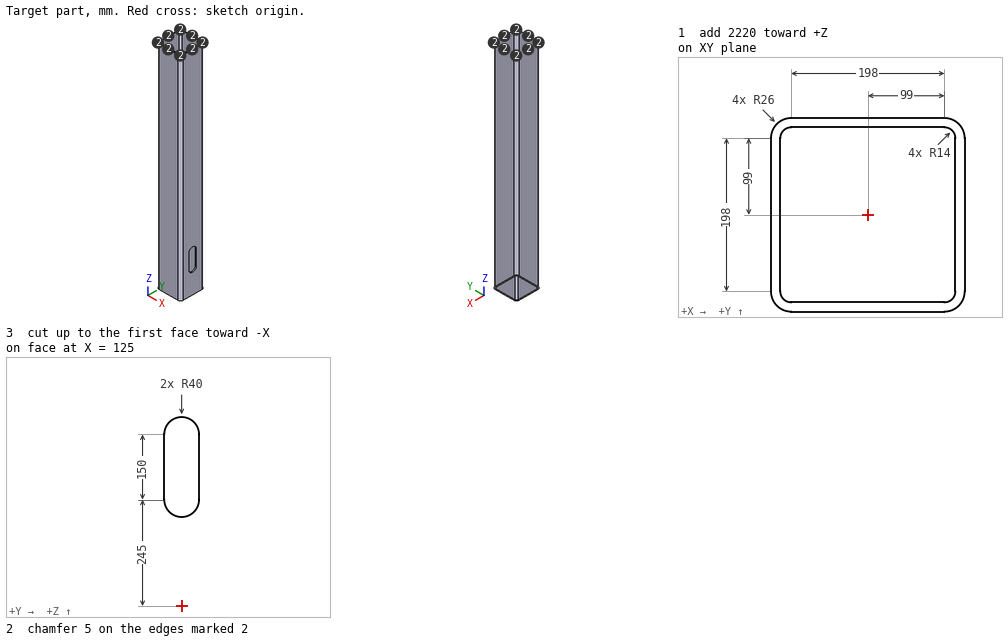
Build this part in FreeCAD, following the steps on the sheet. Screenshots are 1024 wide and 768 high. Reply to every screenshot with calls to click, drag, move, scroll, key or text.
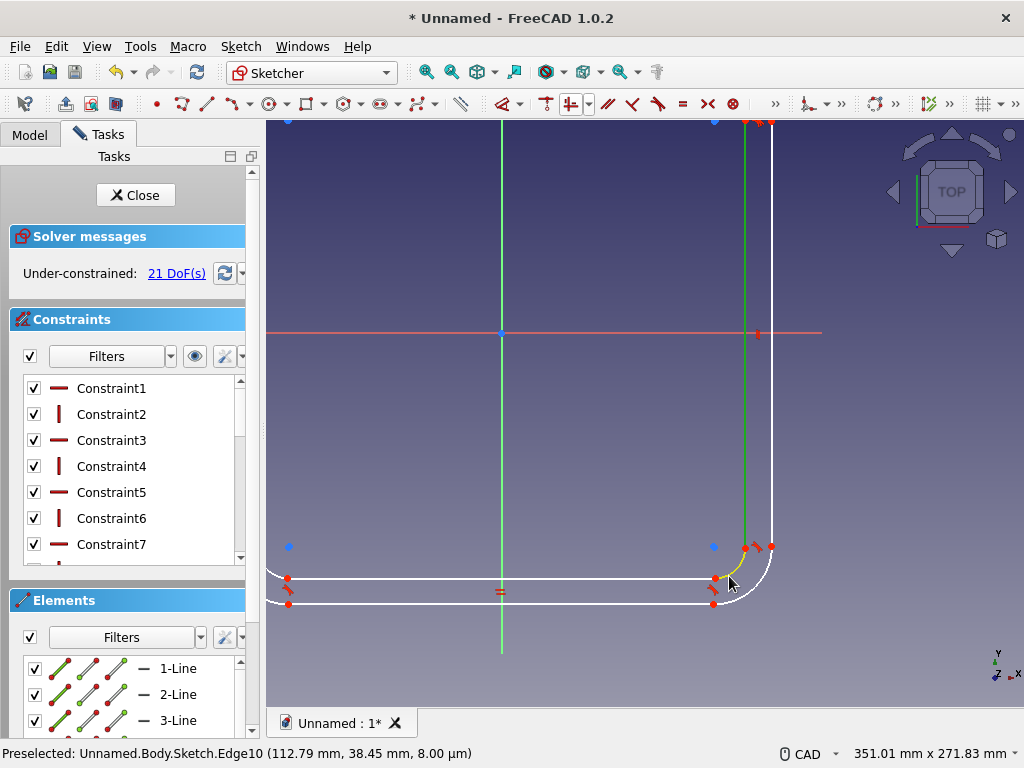
click(729, 575)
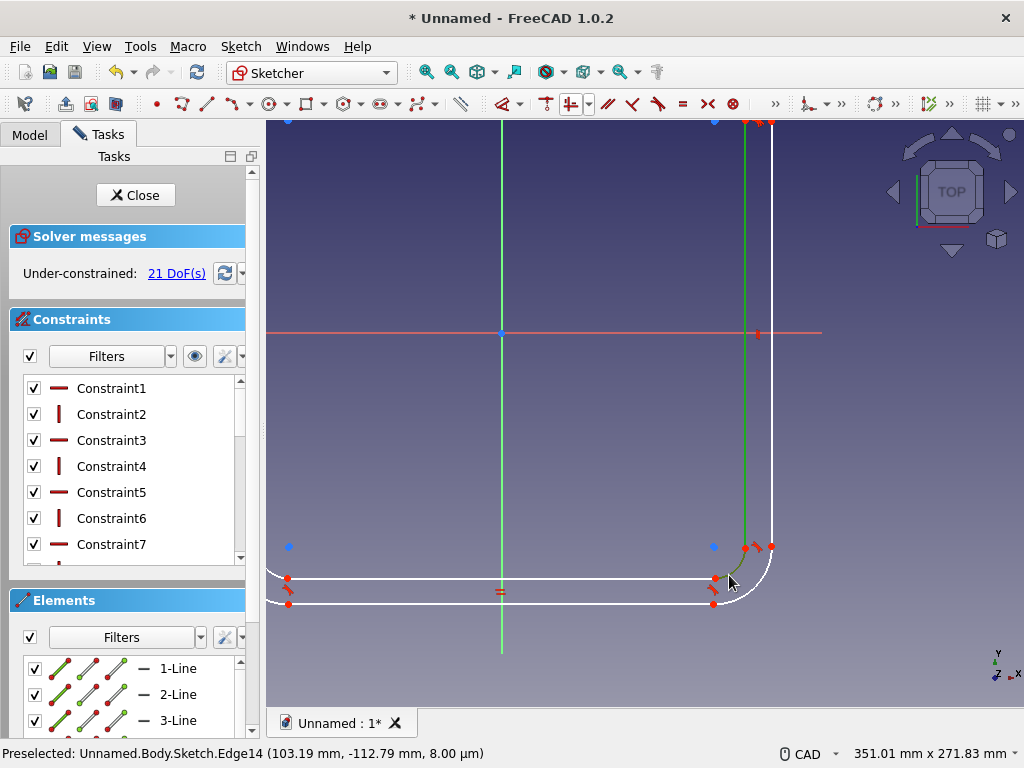
click(658, 104)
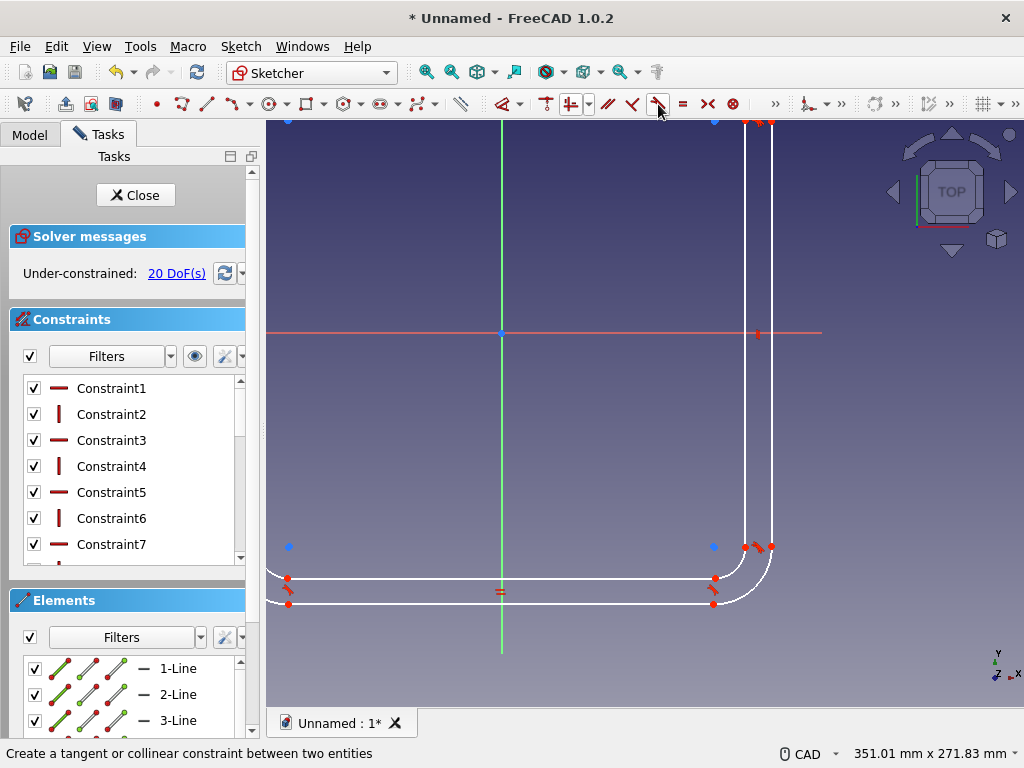
click(587, 579)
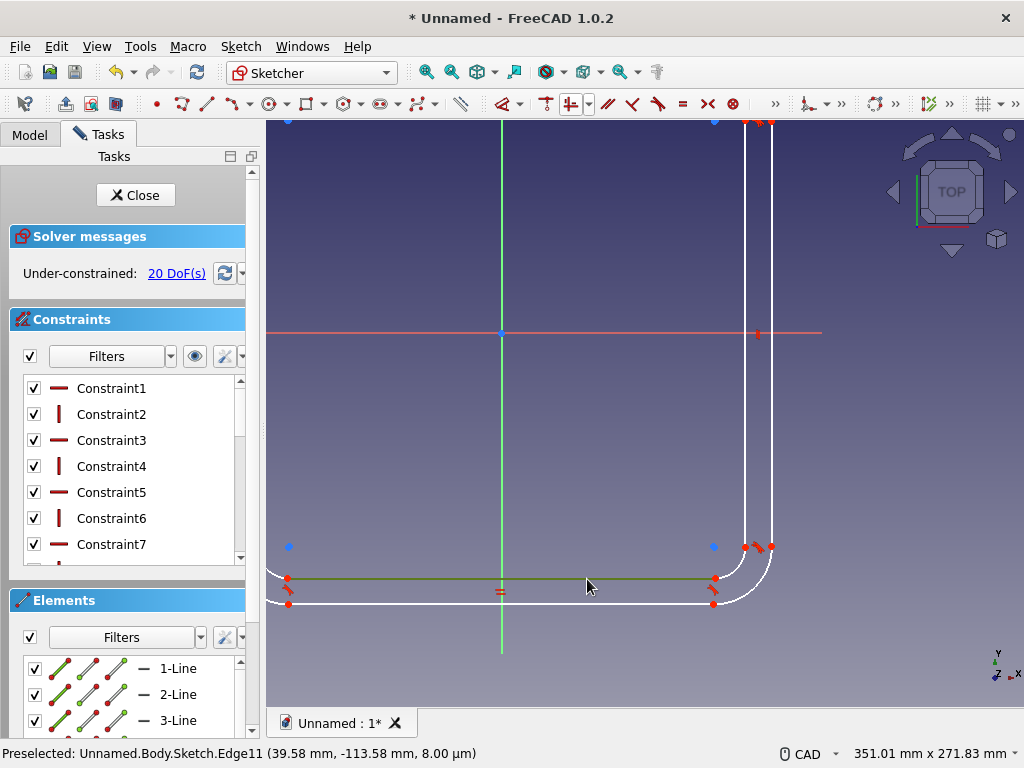
click(729, 575)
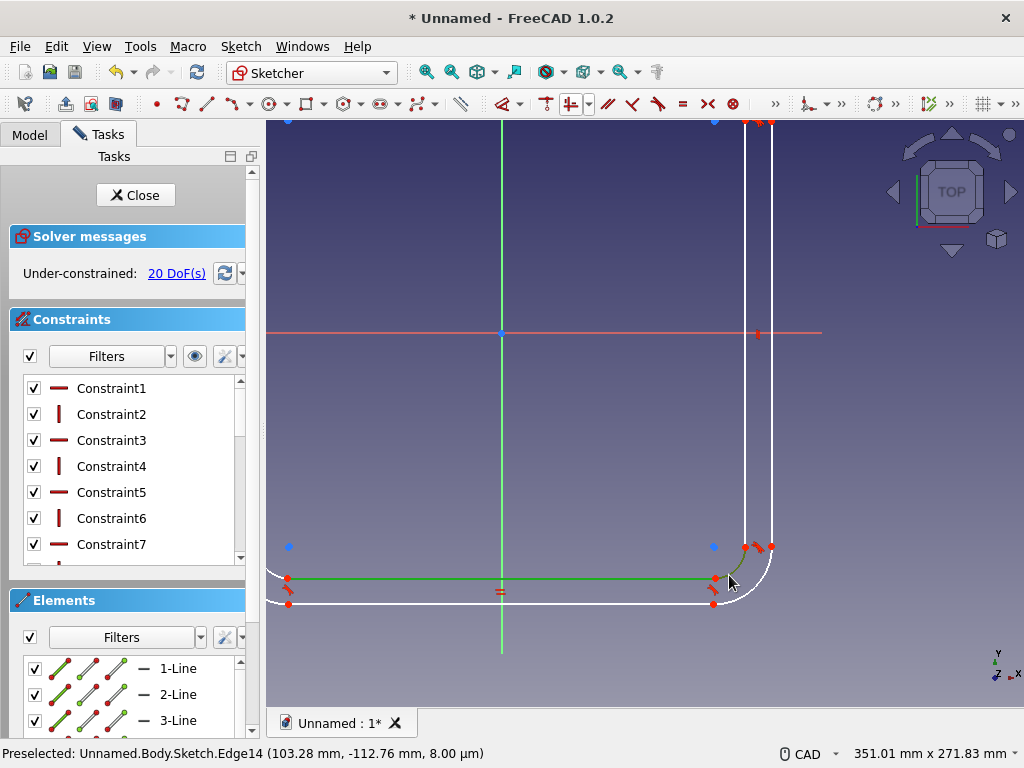
click(658, 104)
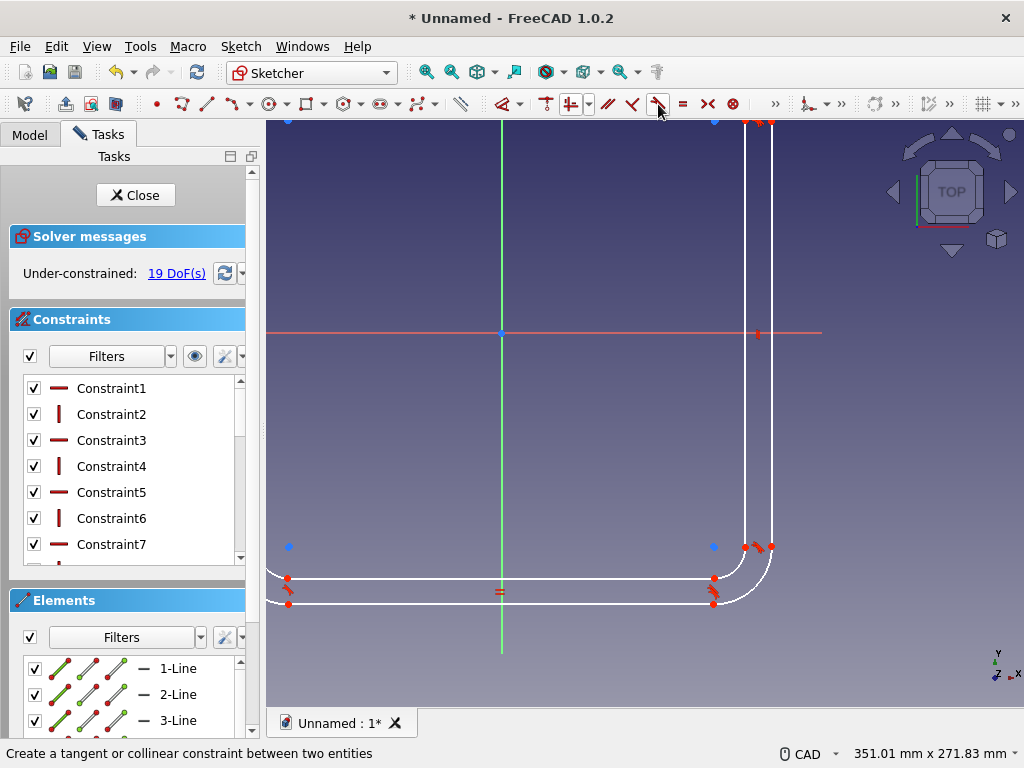
click(586, 579)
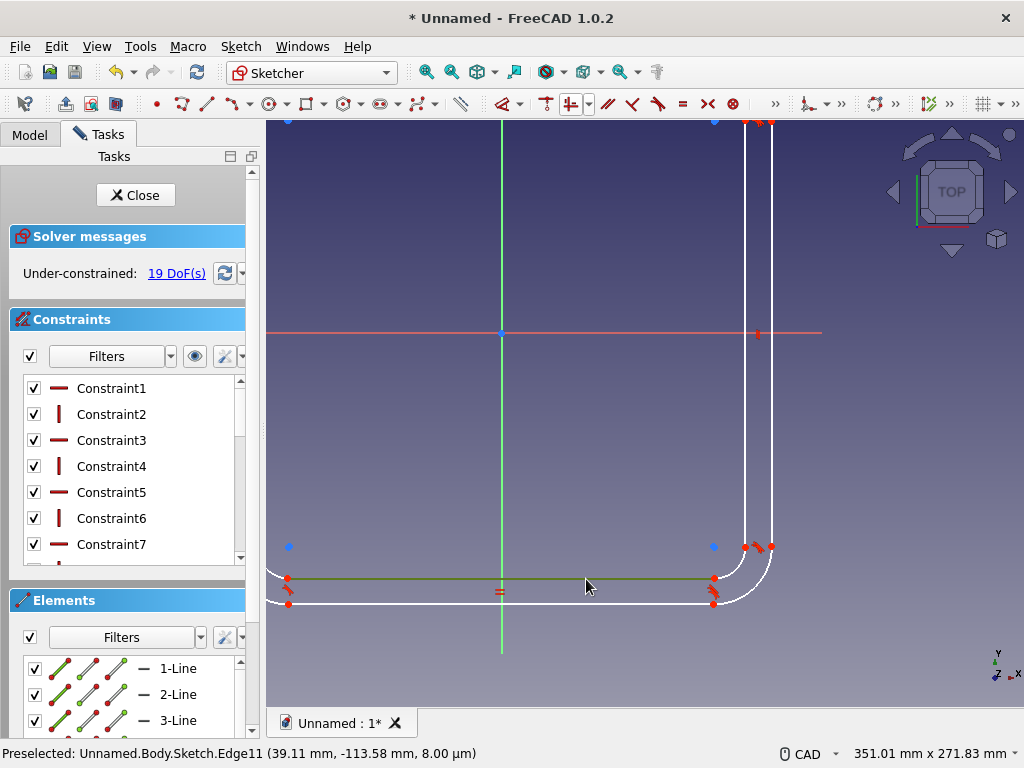
scroll(729, 576, down, 2)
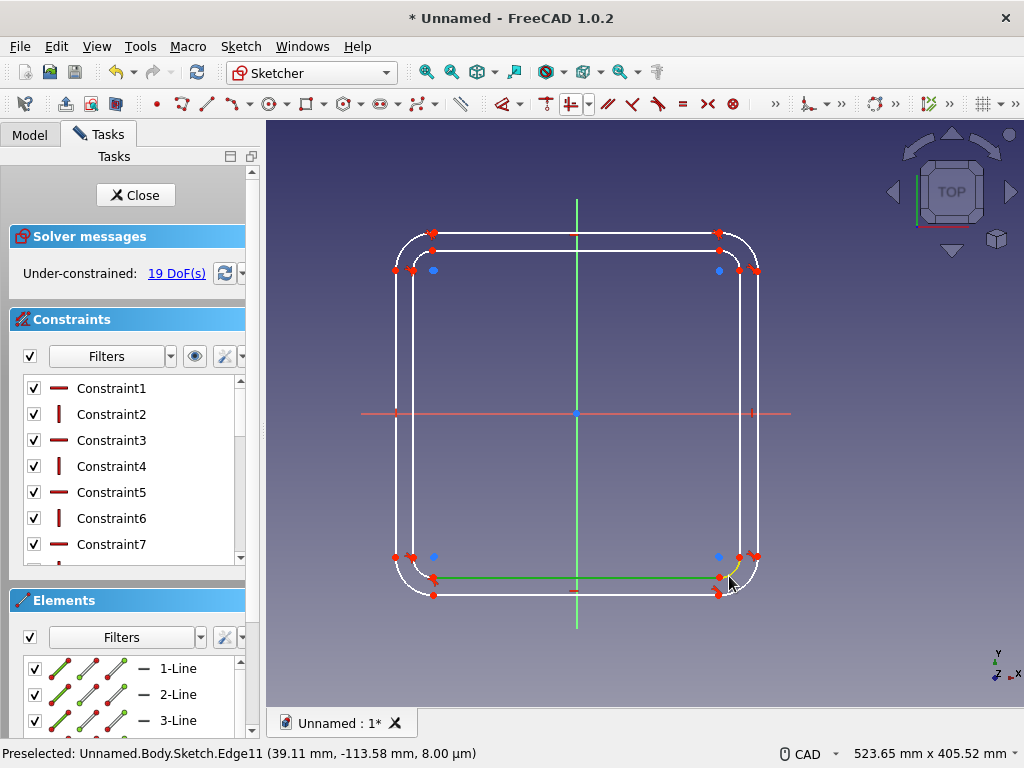
scroll(416, 567, up, 3)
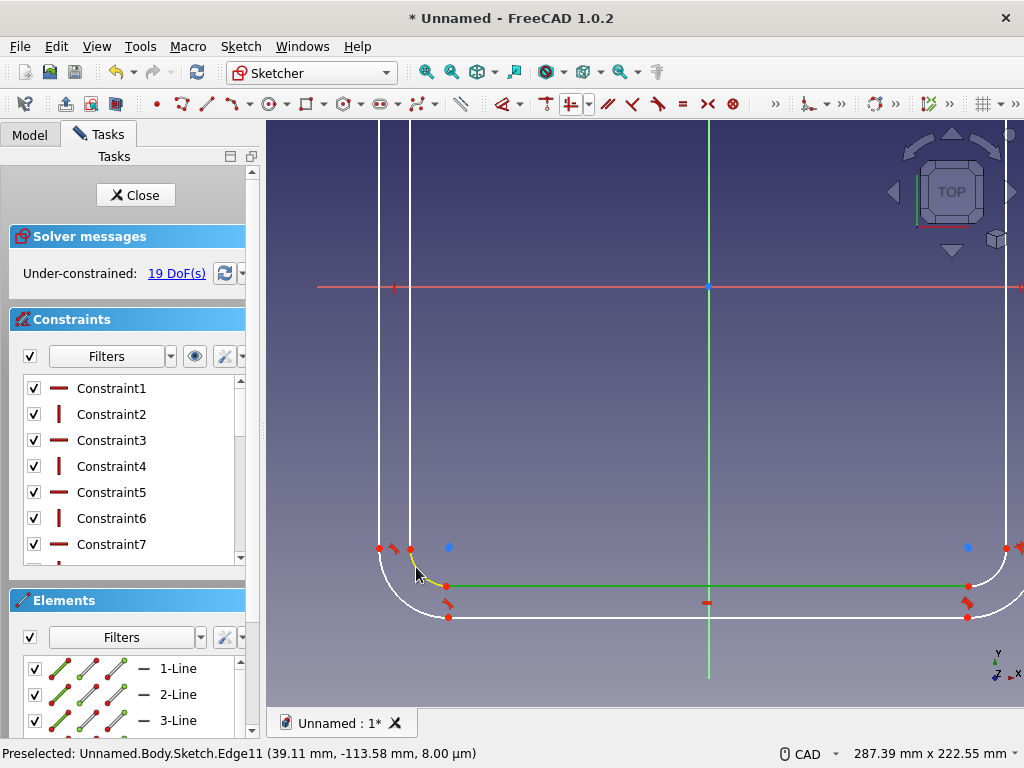
click(415, 566)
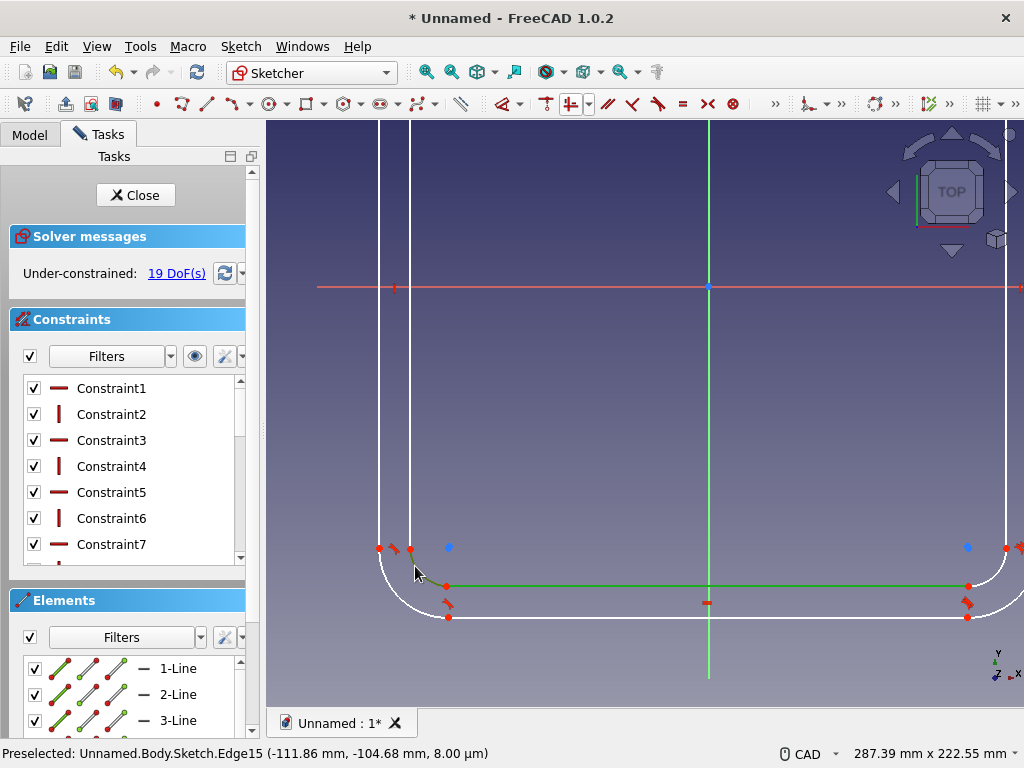
click(658, 104)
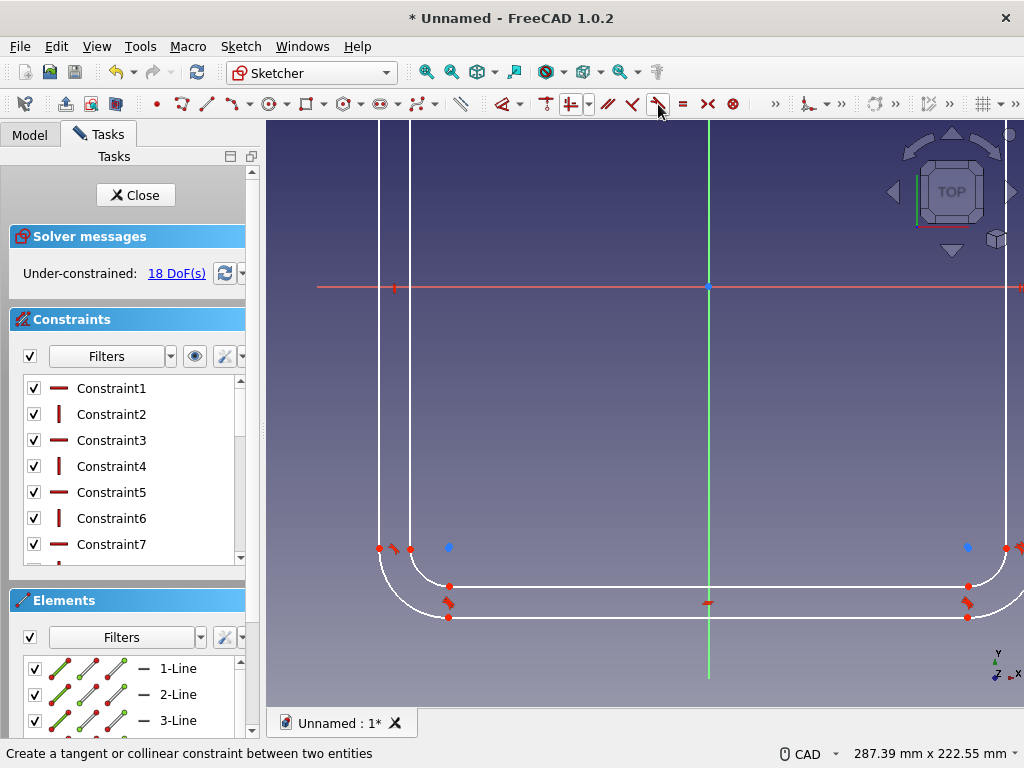
click(410, 393)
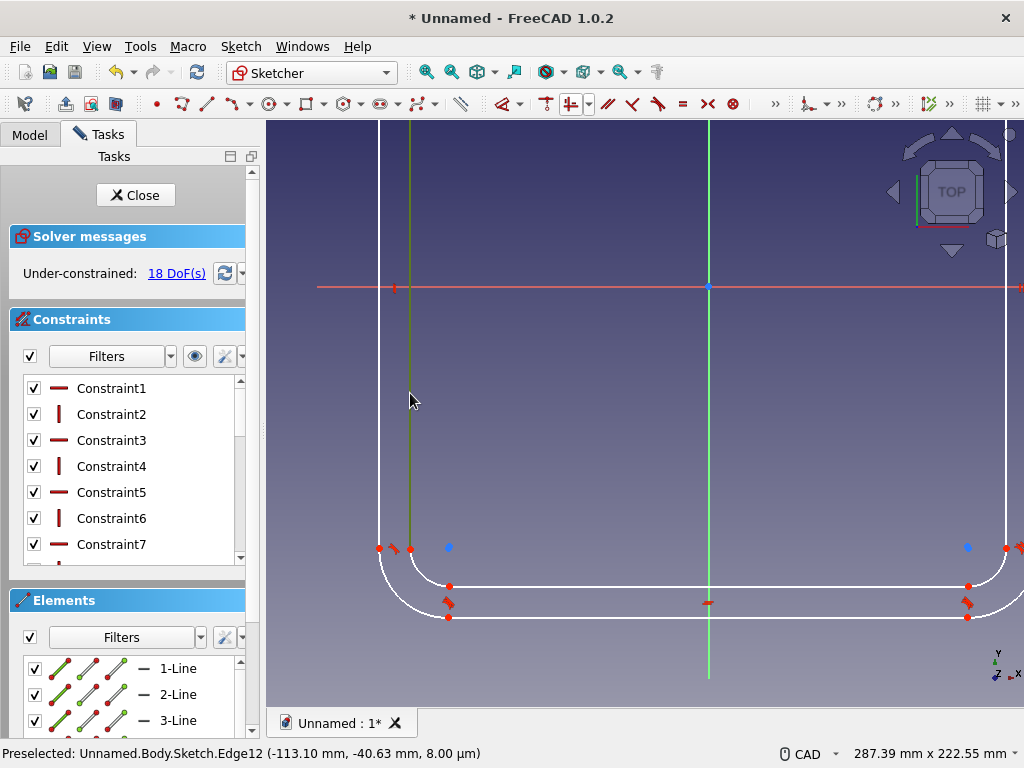
click(416, 567)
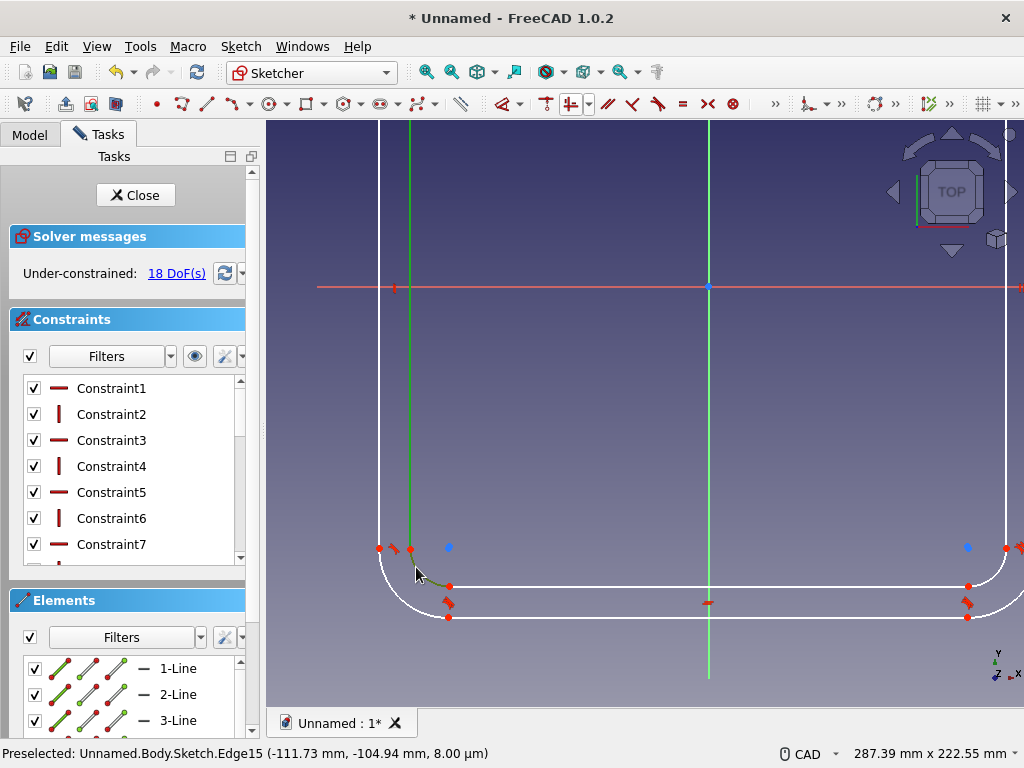
click(658, 104)